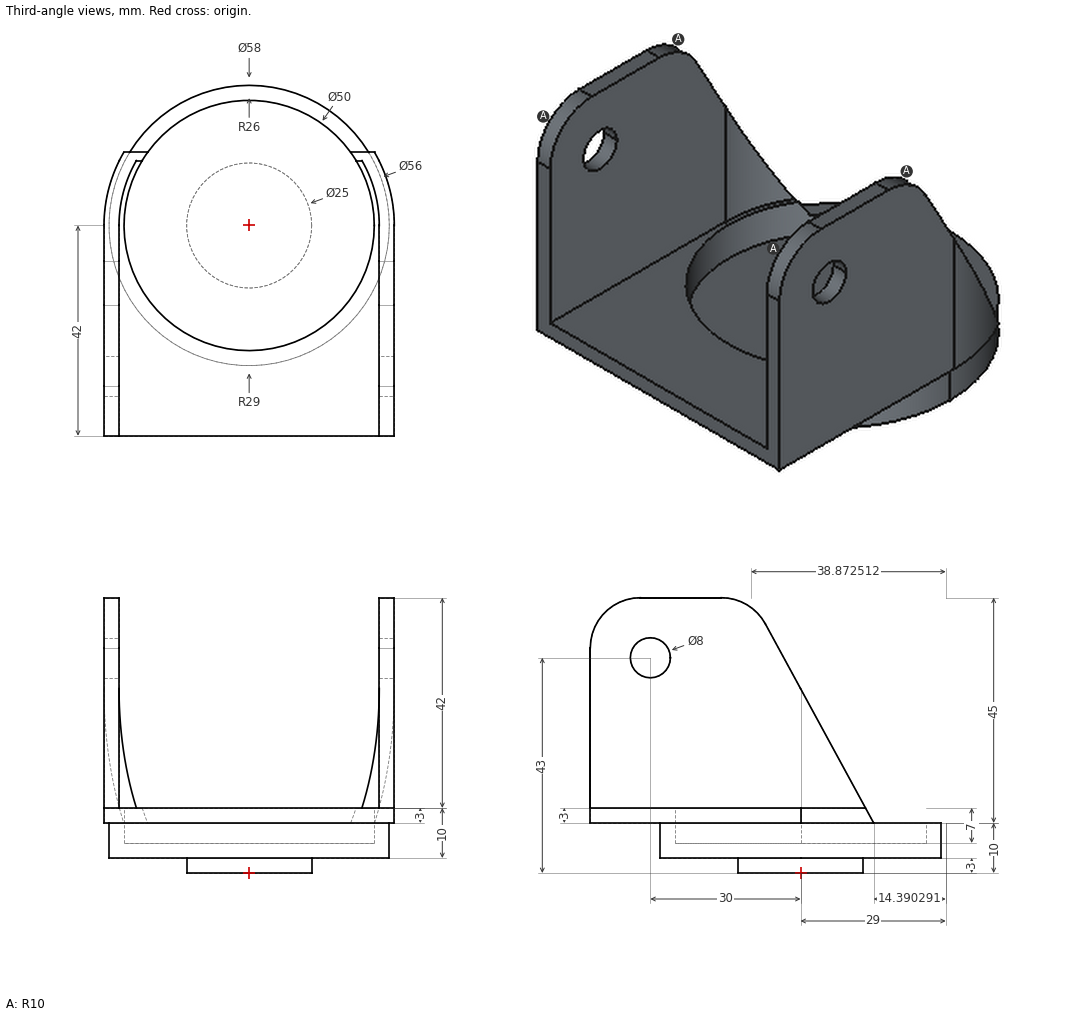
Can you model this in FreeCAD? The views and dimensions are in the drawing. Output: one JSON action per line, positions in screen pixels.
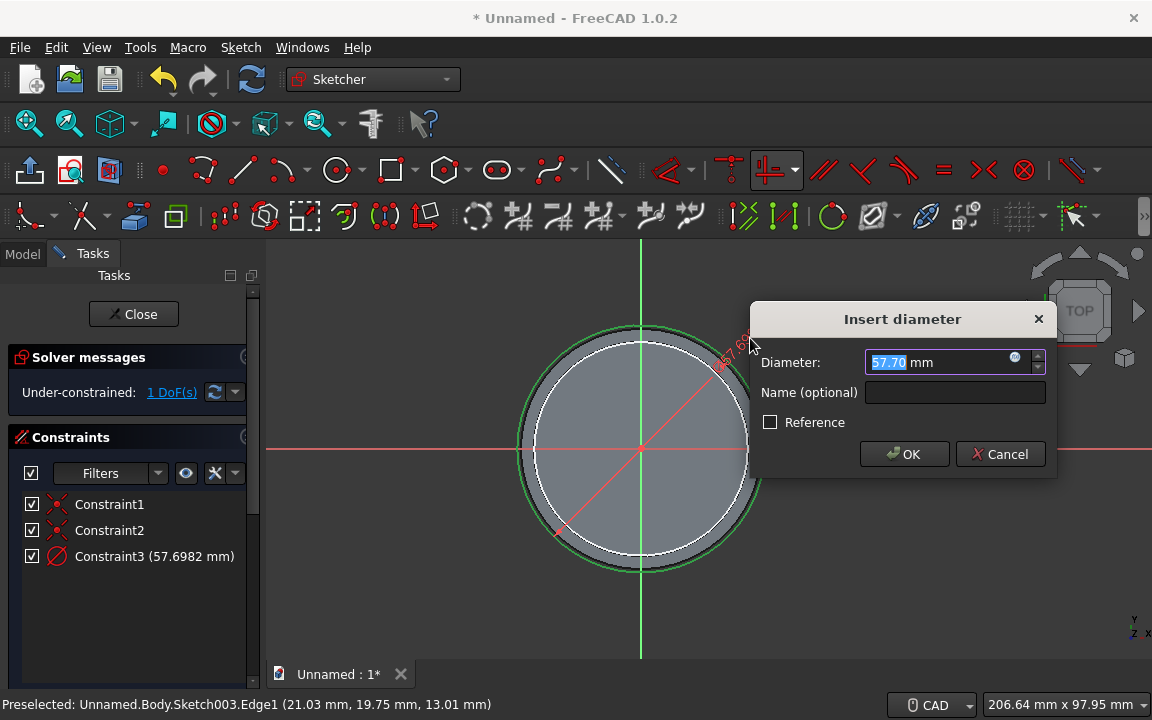
{"action": "type", "text": "58"}
{"action": "key", "text": "Return"}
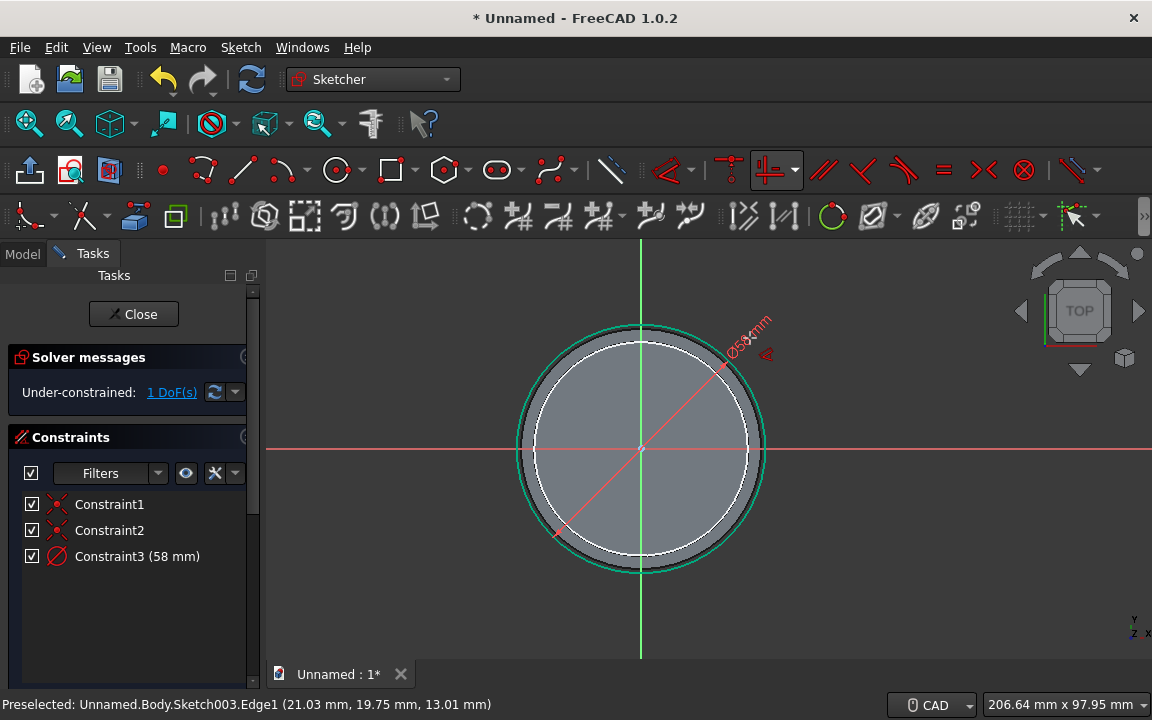
{"action": "left_click", "coordinate": [716, 373]}
{"action": "left_click", "coordinate": [774, 409]}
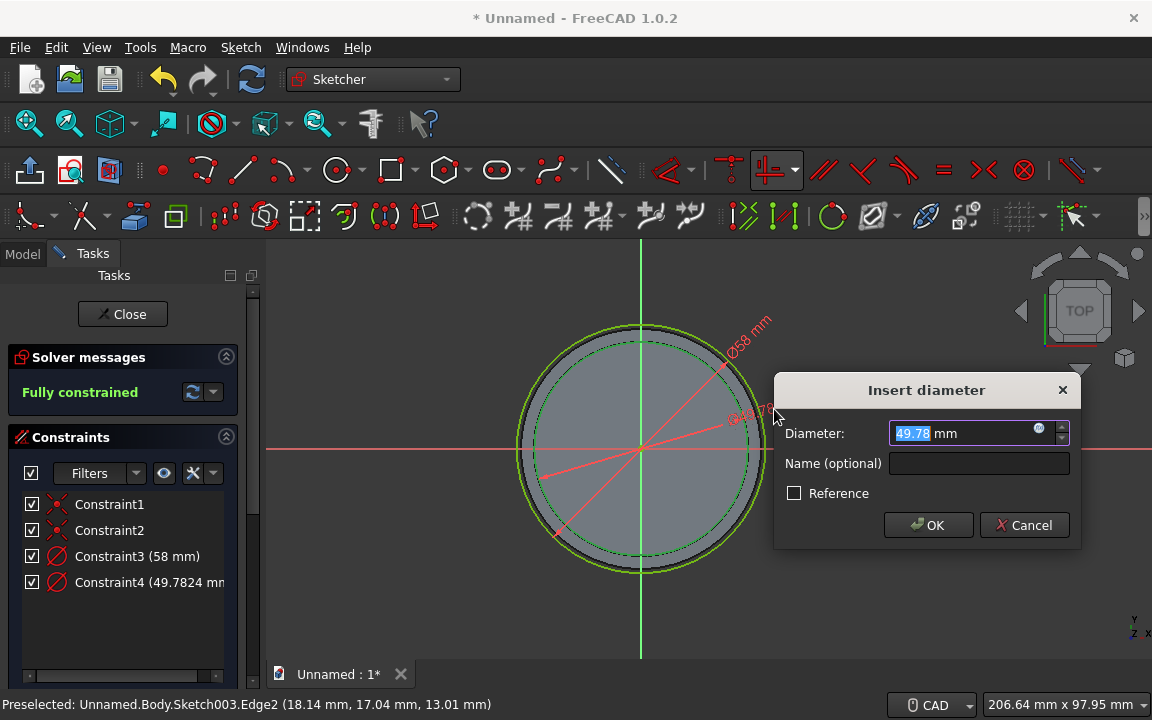
{"action": "type", "text": "50"}
{"action": "key", "text": "Return"}
{"action": "key", "text": "Escape"}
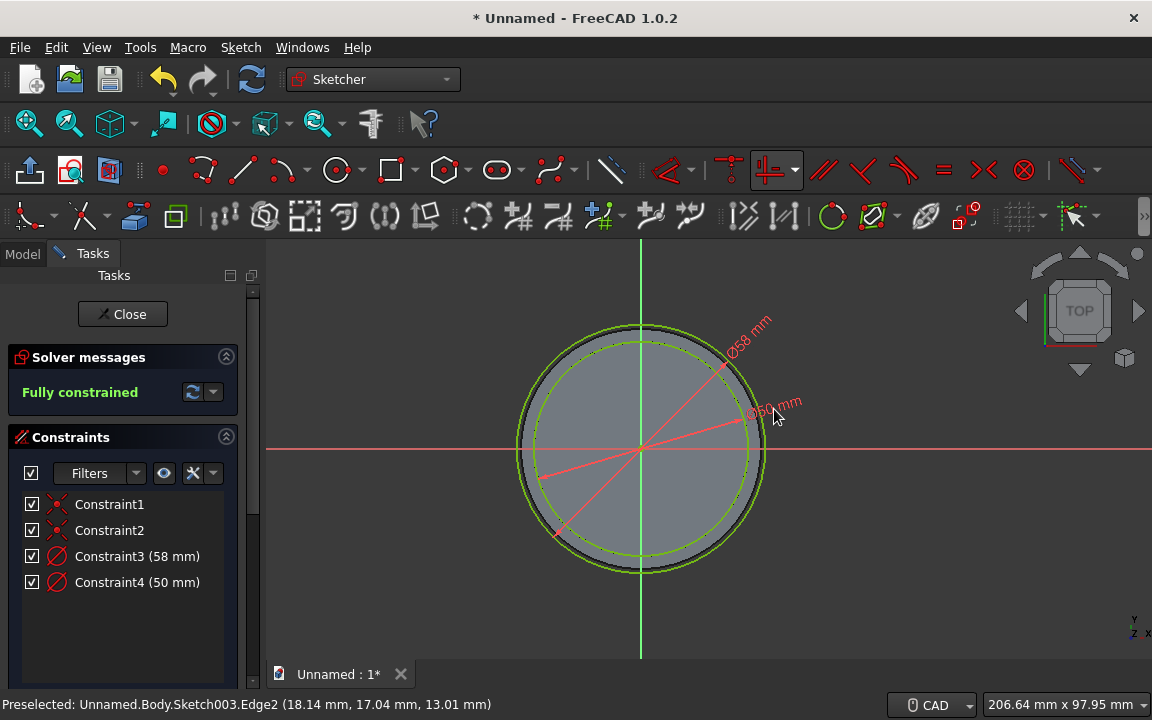
{"action": "left_click", "coordinate": [123, 314]}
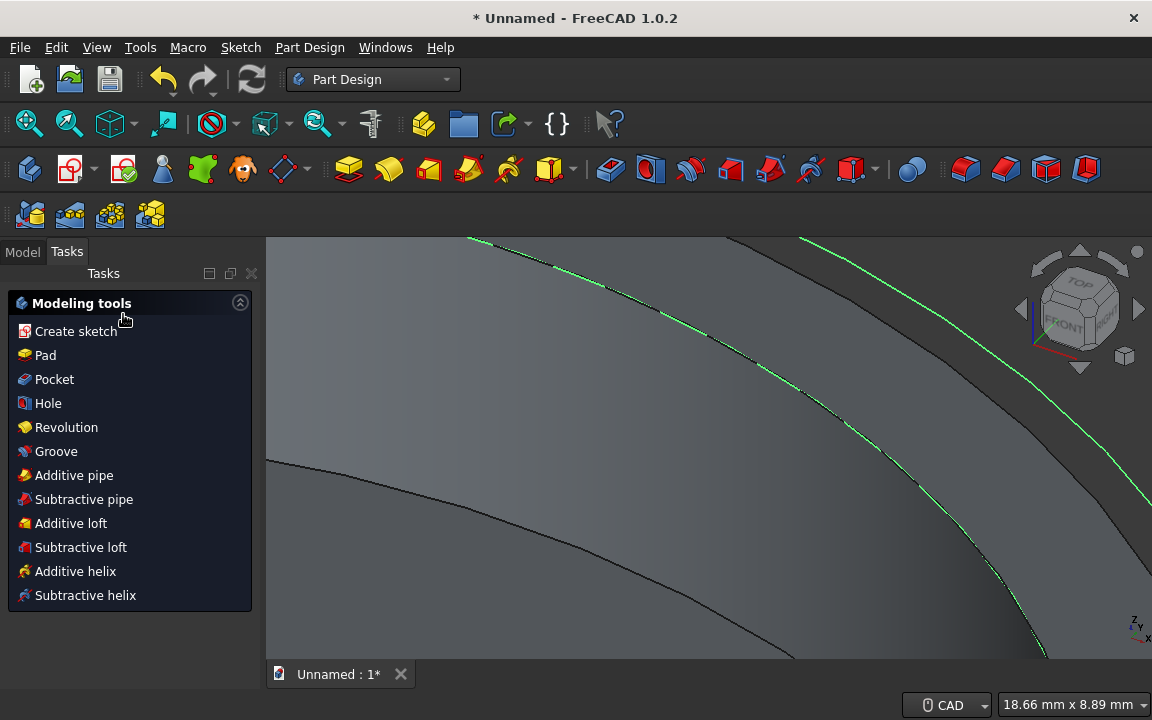
{"action": "left_click", "coordinate": [350, 170]}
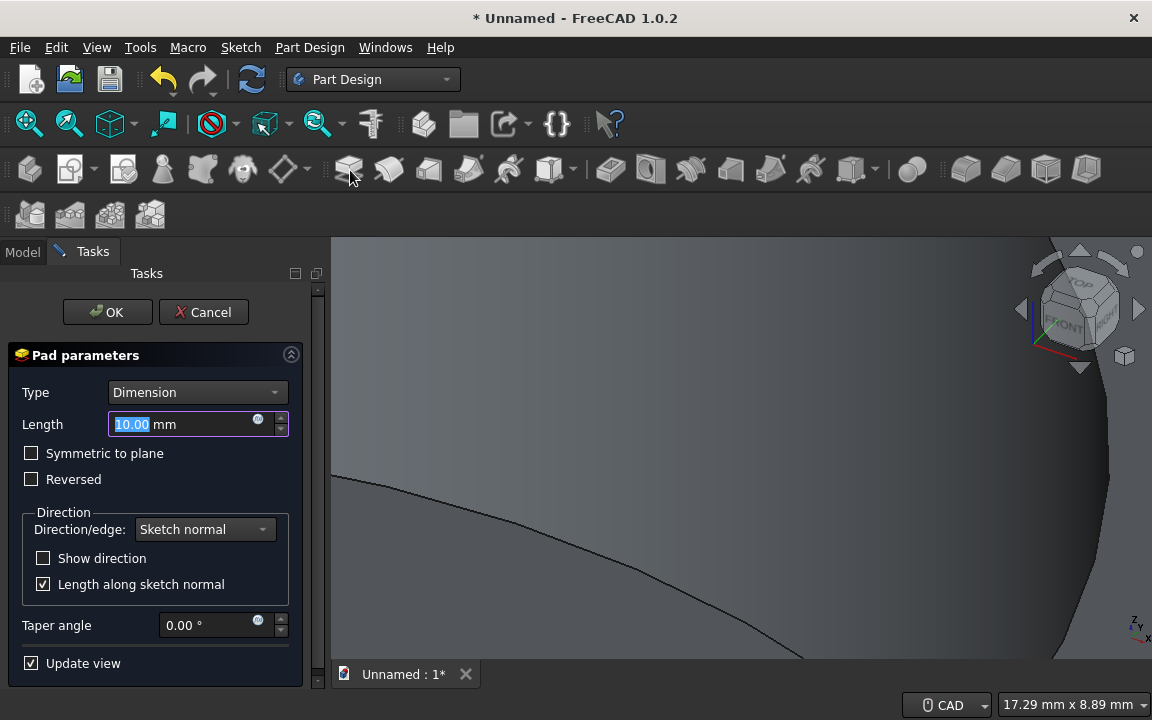
{"action": "type", "text": "3"}
{"action": "key", "text": "Tab"}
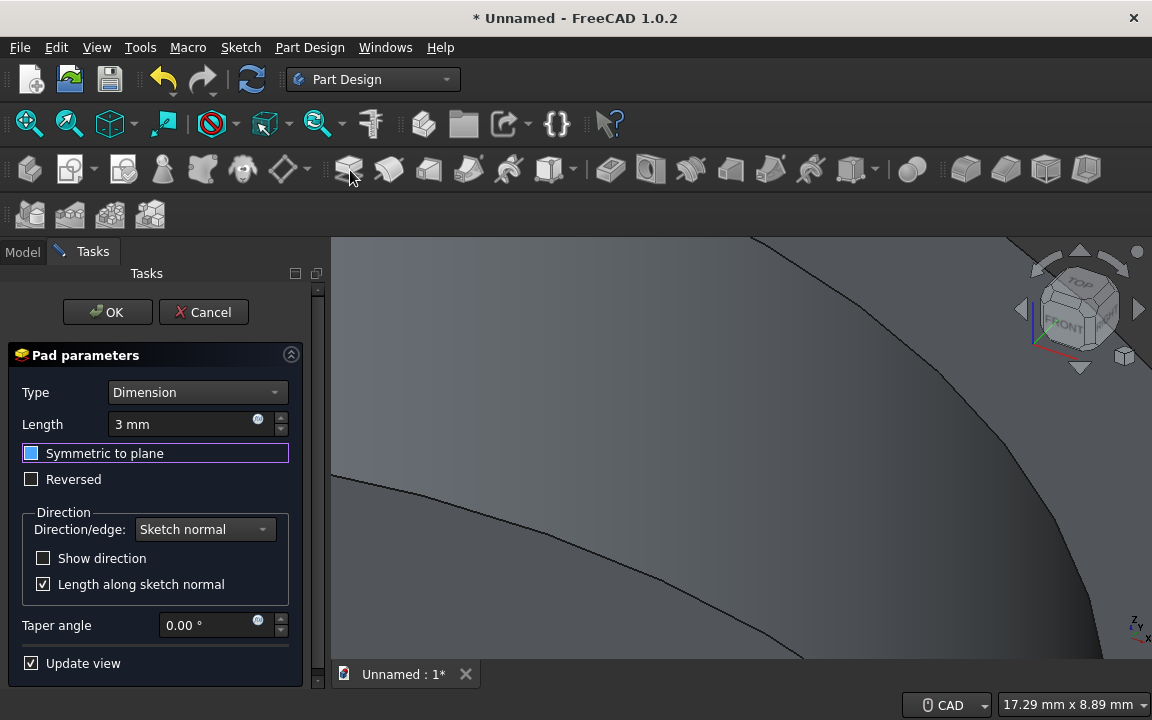
{"action": "left_click", "coordinate": [30, 479]}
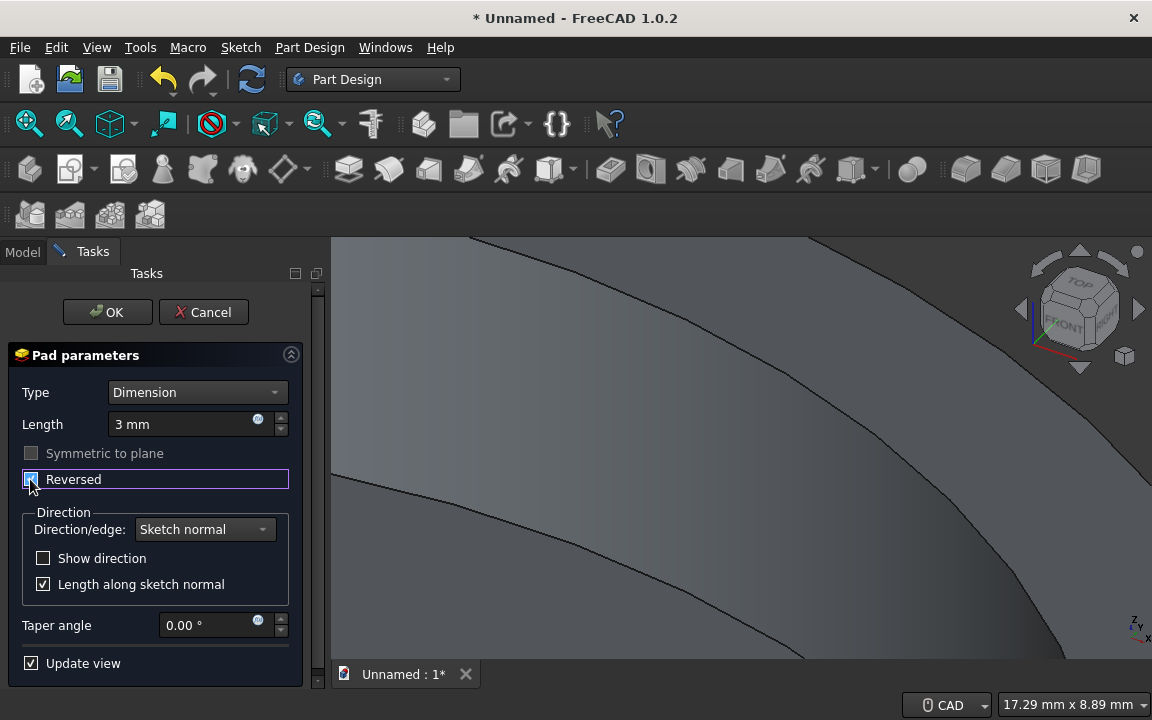
{"action": "left_click", "coordinate": [108, 312]}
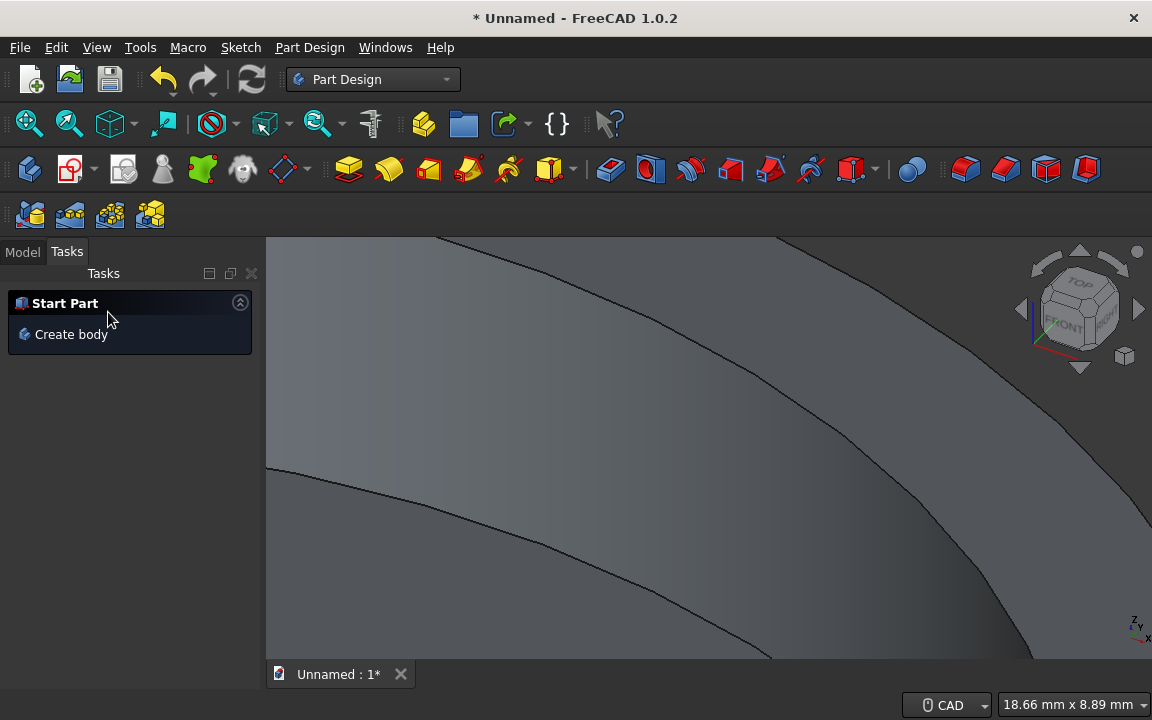
{"action": "left_click", "coordinate": [30, 124]}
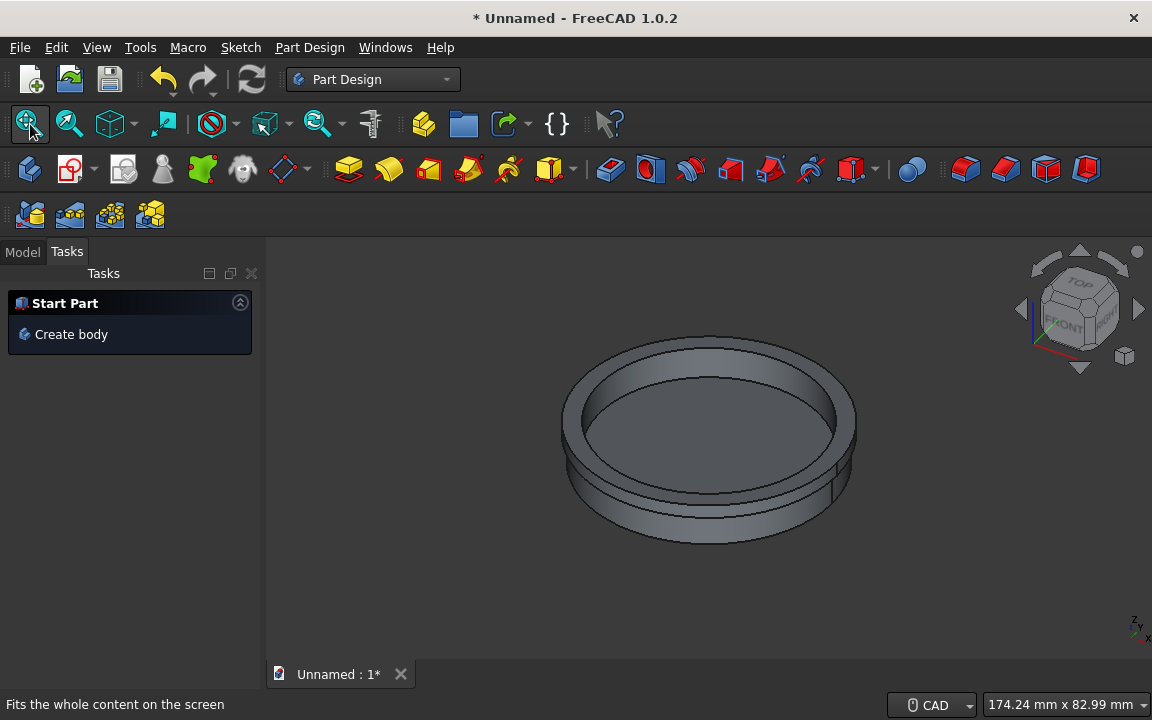
{"action": "left_click", "coordinate": [609, 471]}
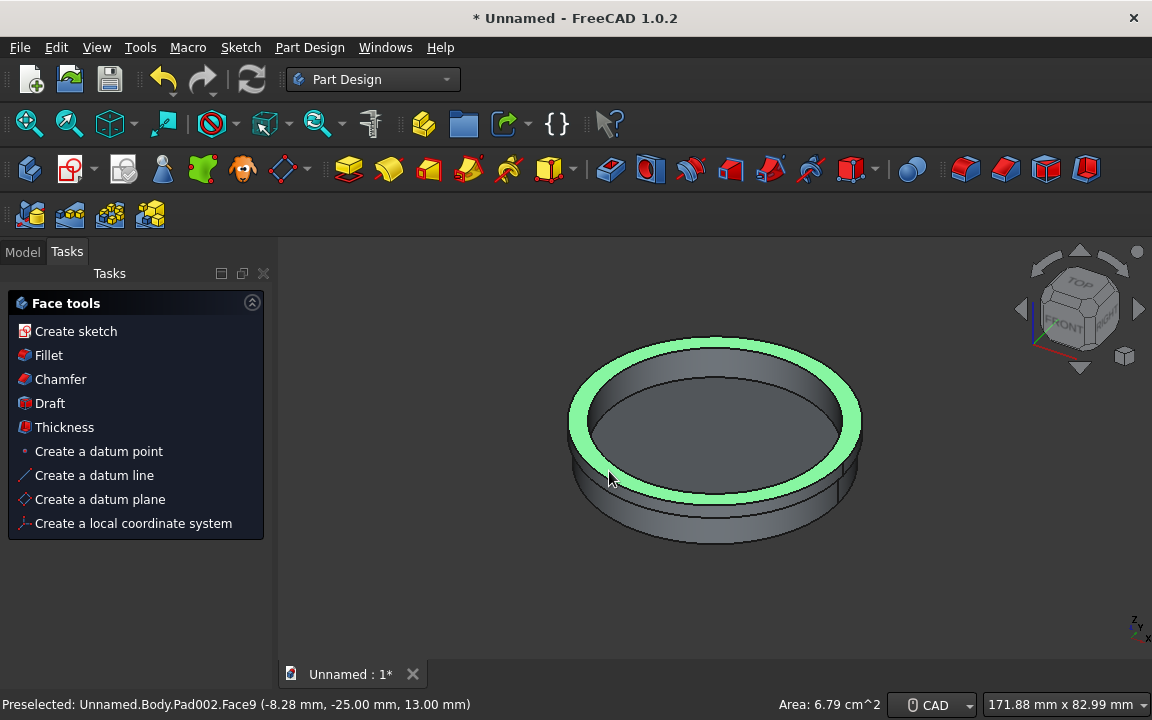
{"action": "left_click", "coordinate": [70, 170]}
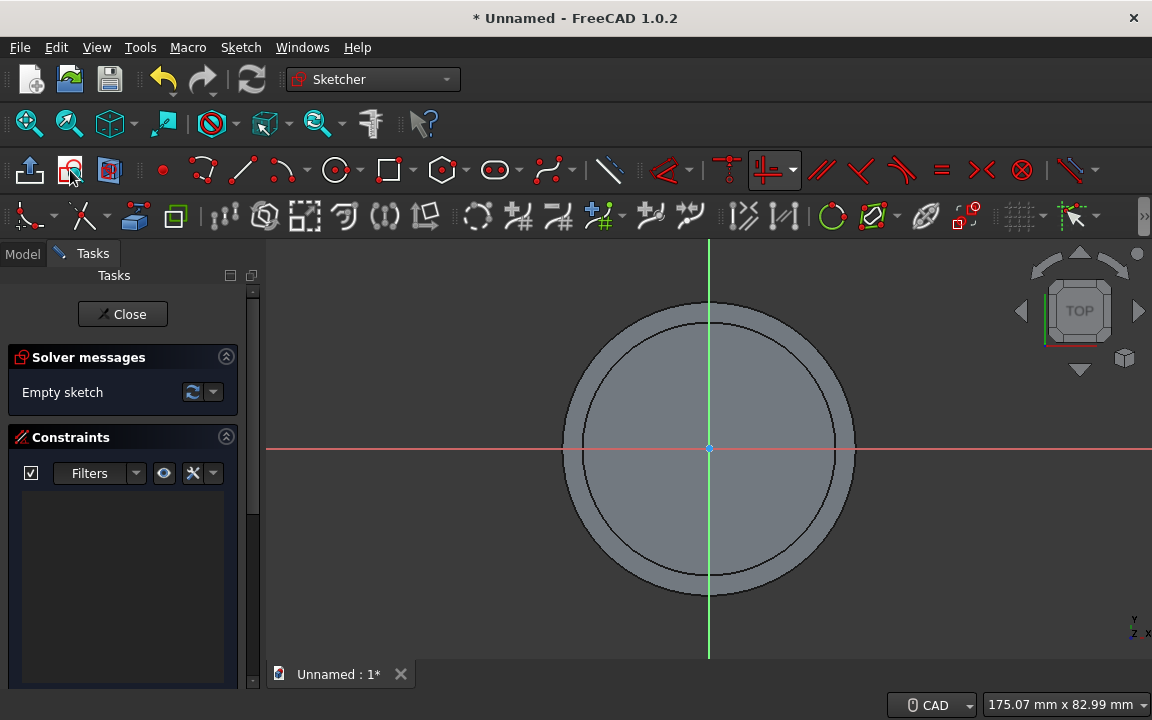
{"action": "scroll", "coordinate": [331, 267], "scroll_direction": "down", "scroll_amount": 1}